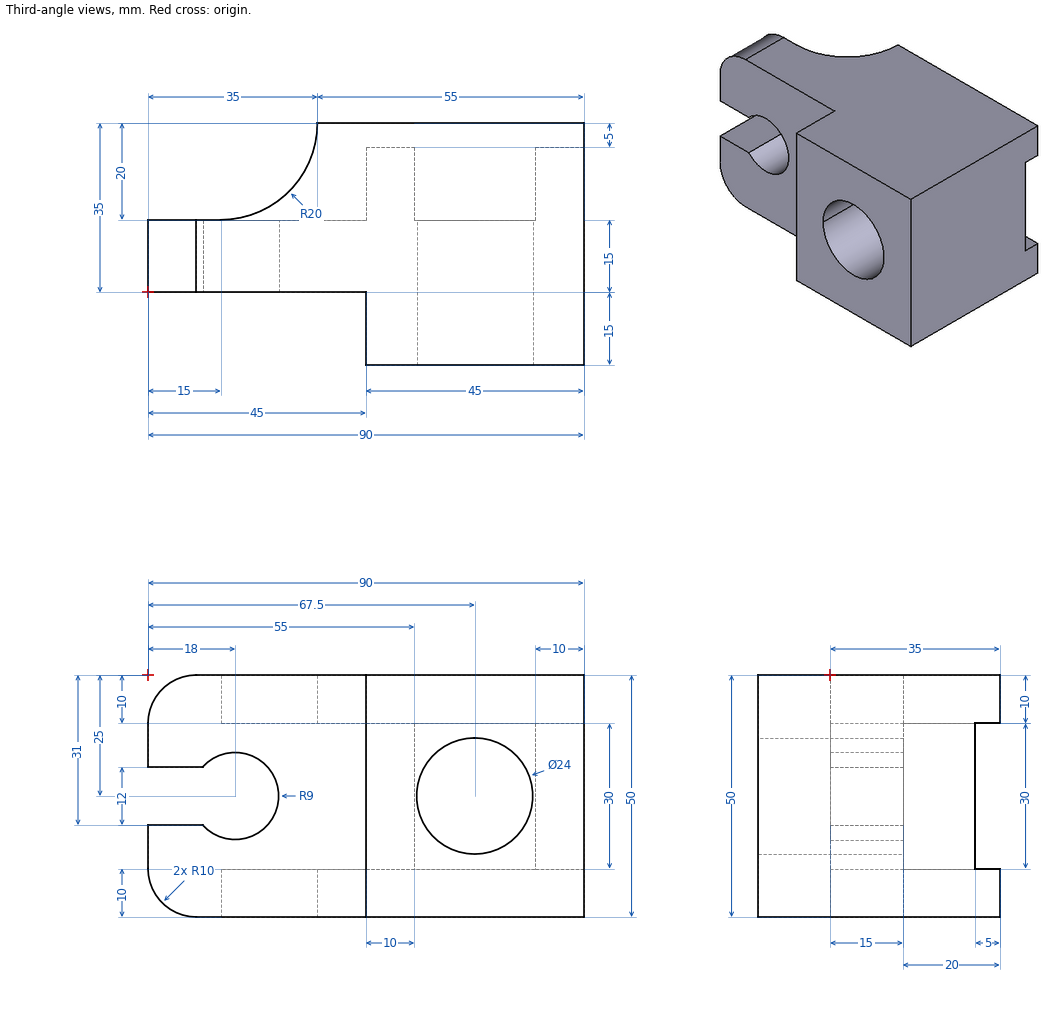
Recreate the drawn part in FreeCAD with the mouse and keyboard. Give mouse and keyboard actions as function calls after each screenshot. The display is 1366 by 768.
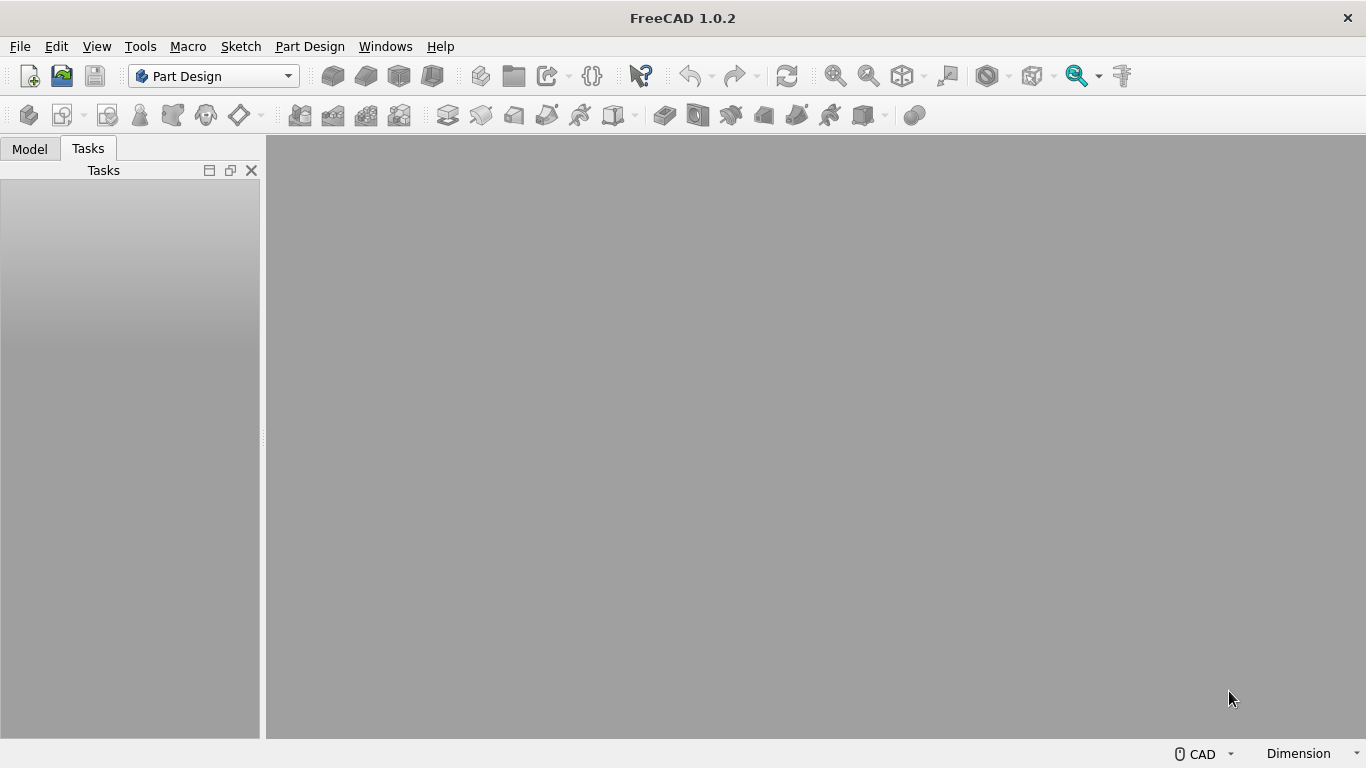
click(29, 76)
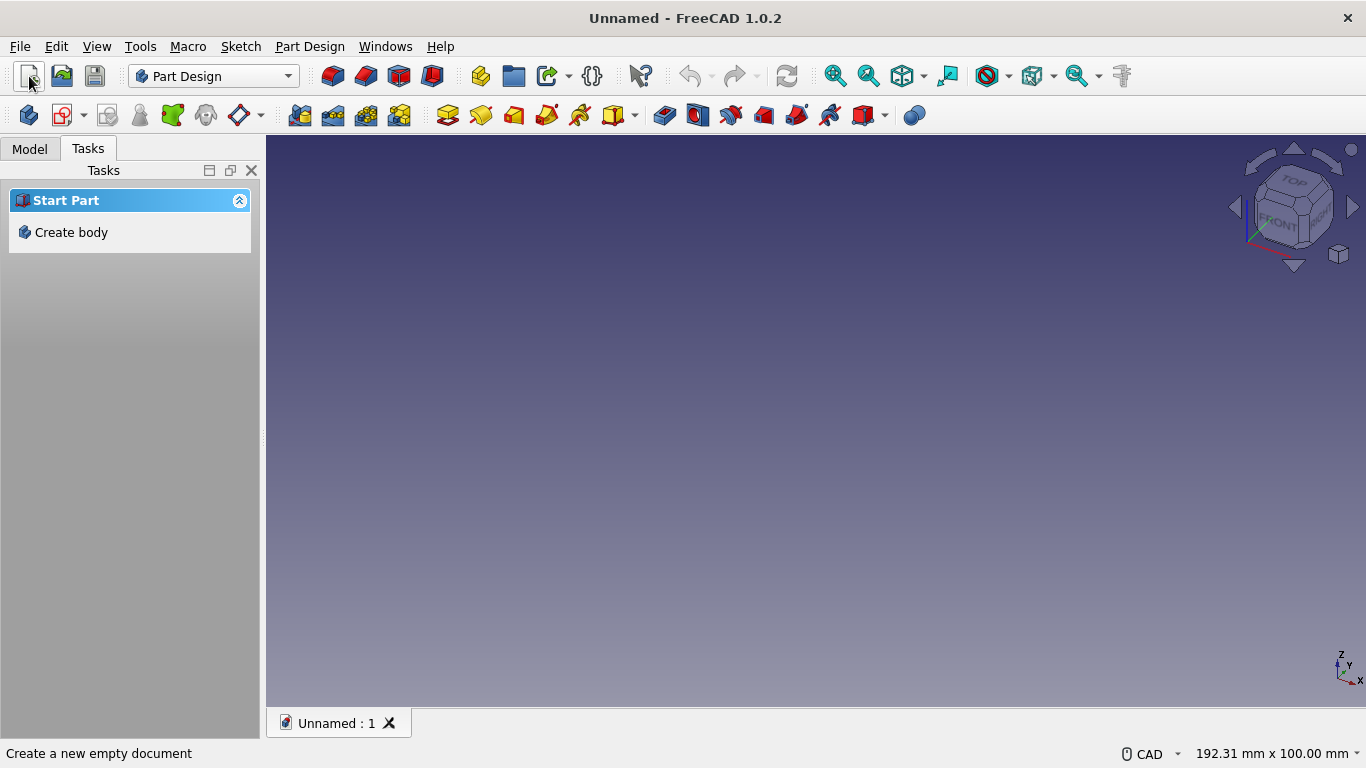
click(62, 116)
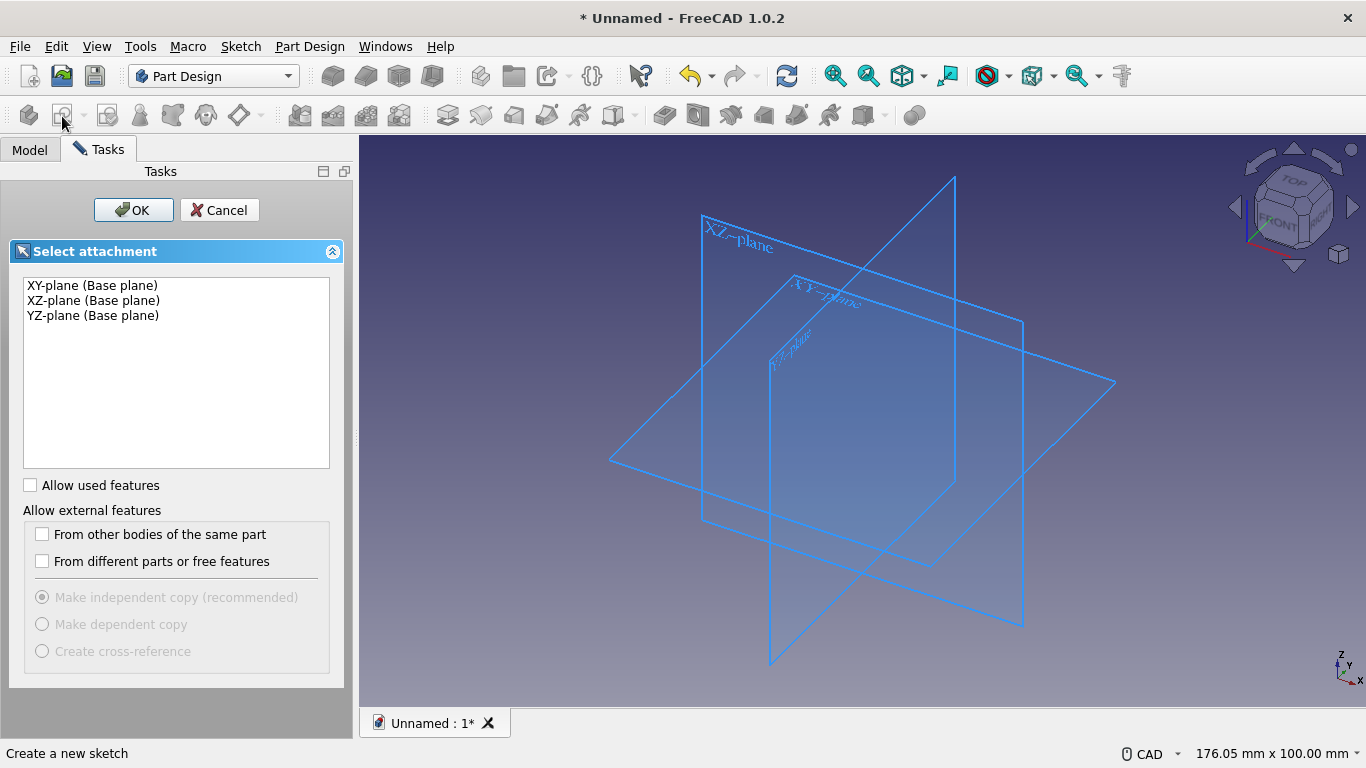
click(84, 286)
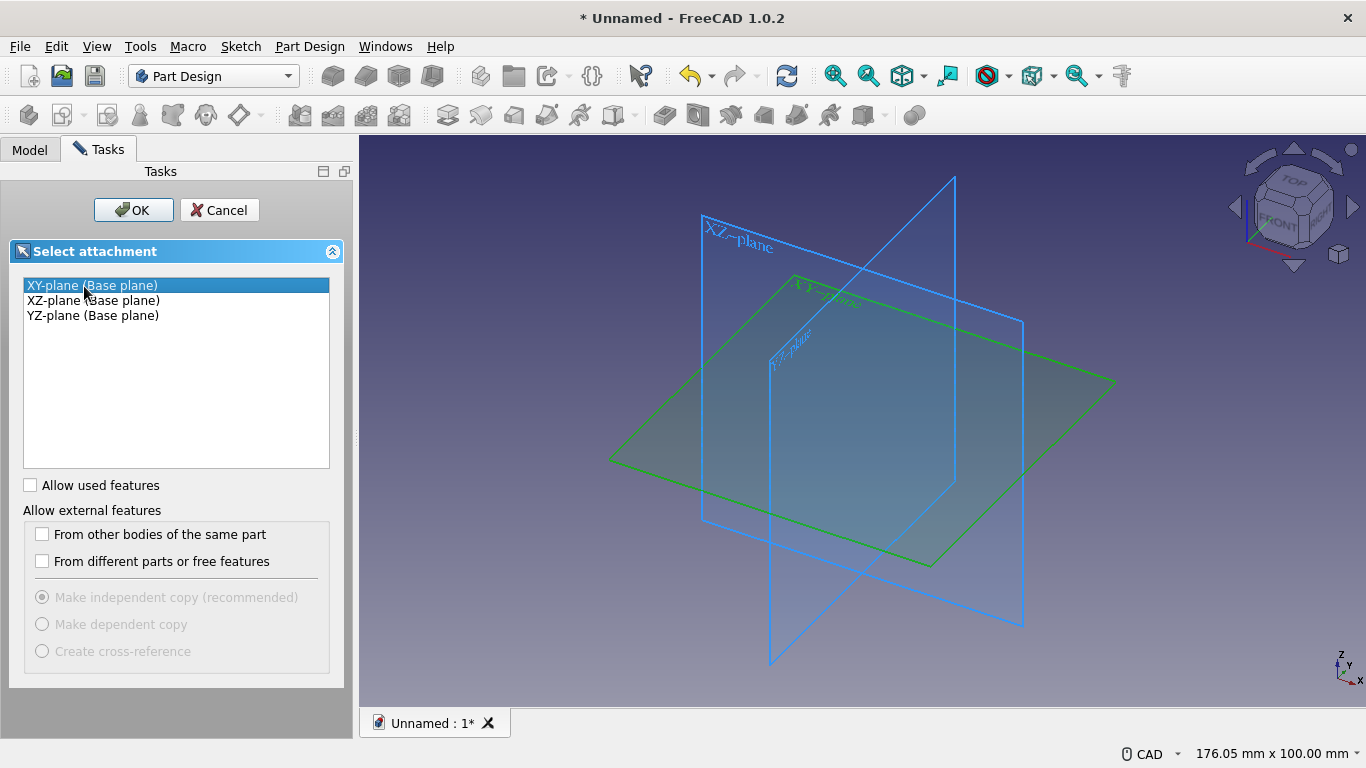
click(134, 210)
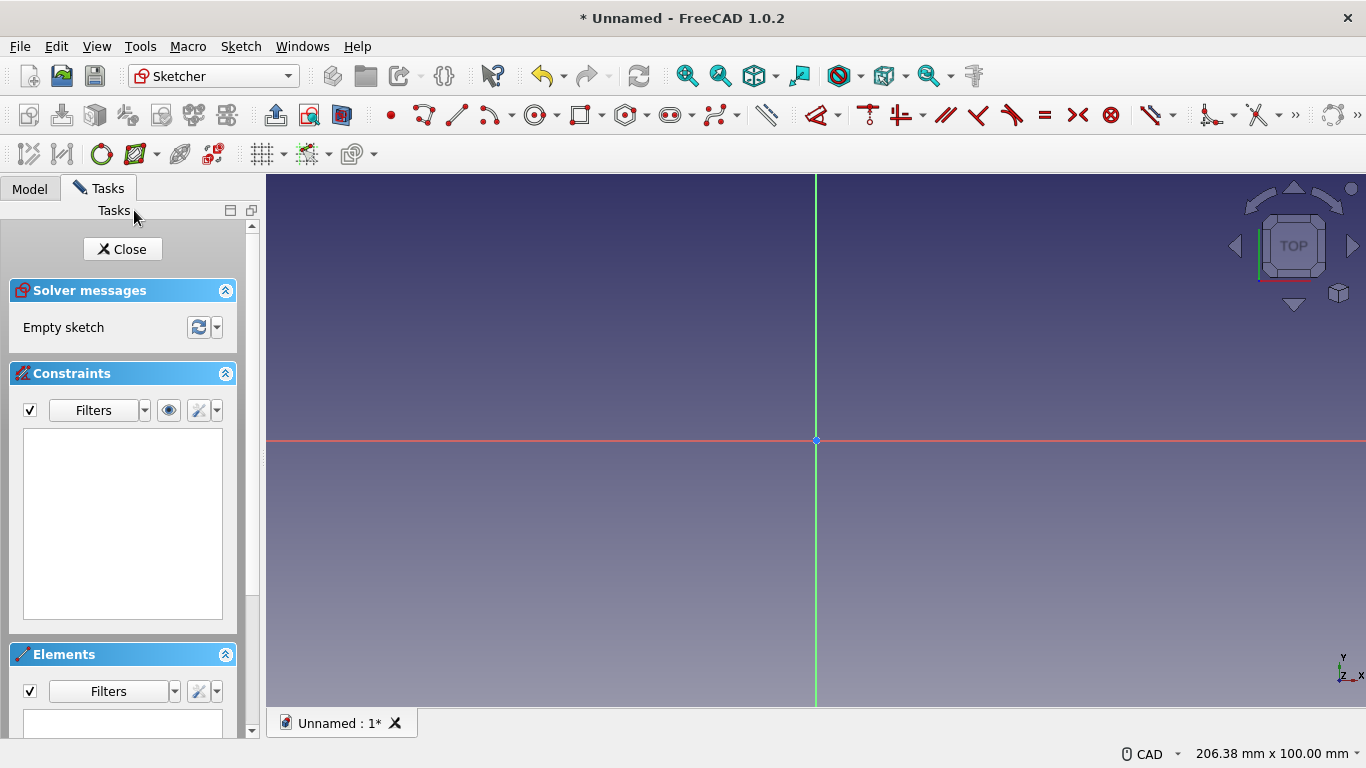
scroll(294, 621, down, 1)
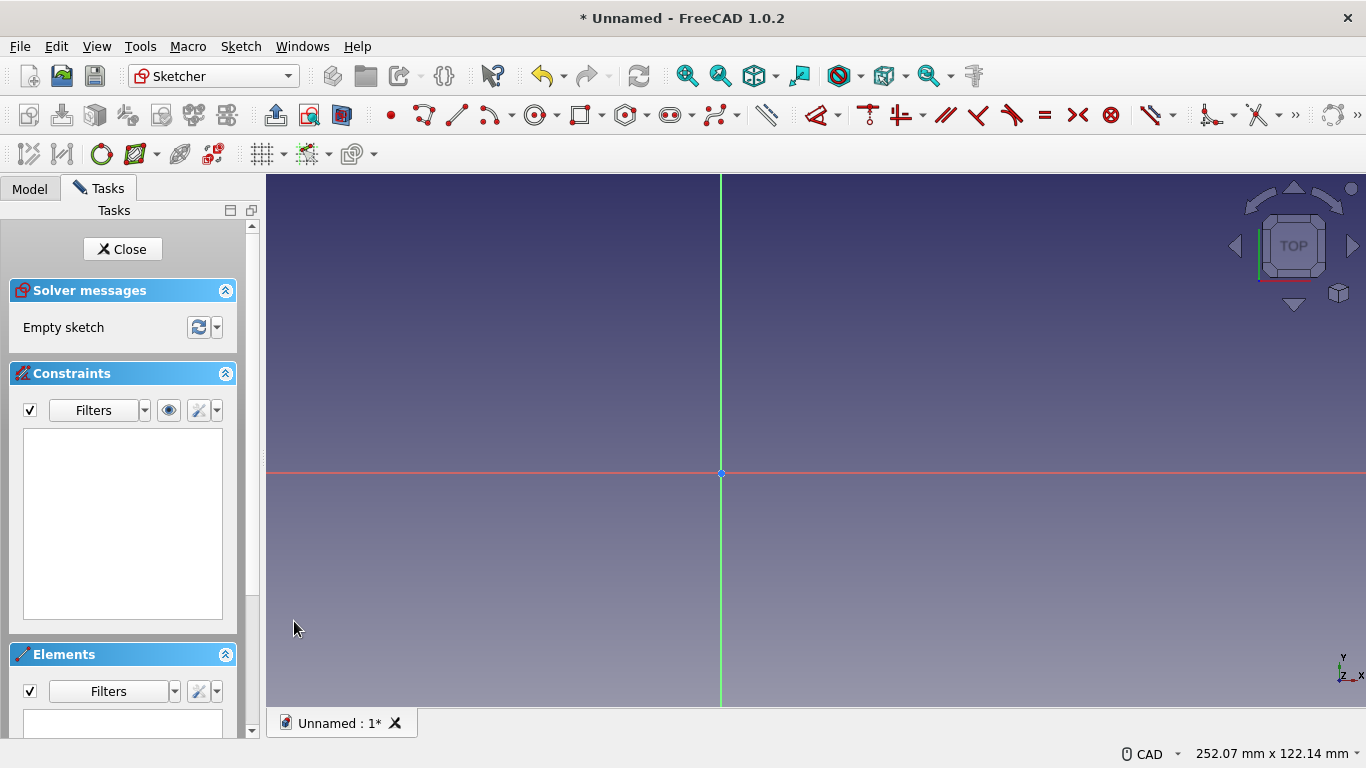
scroll(1201, 441, up, 2)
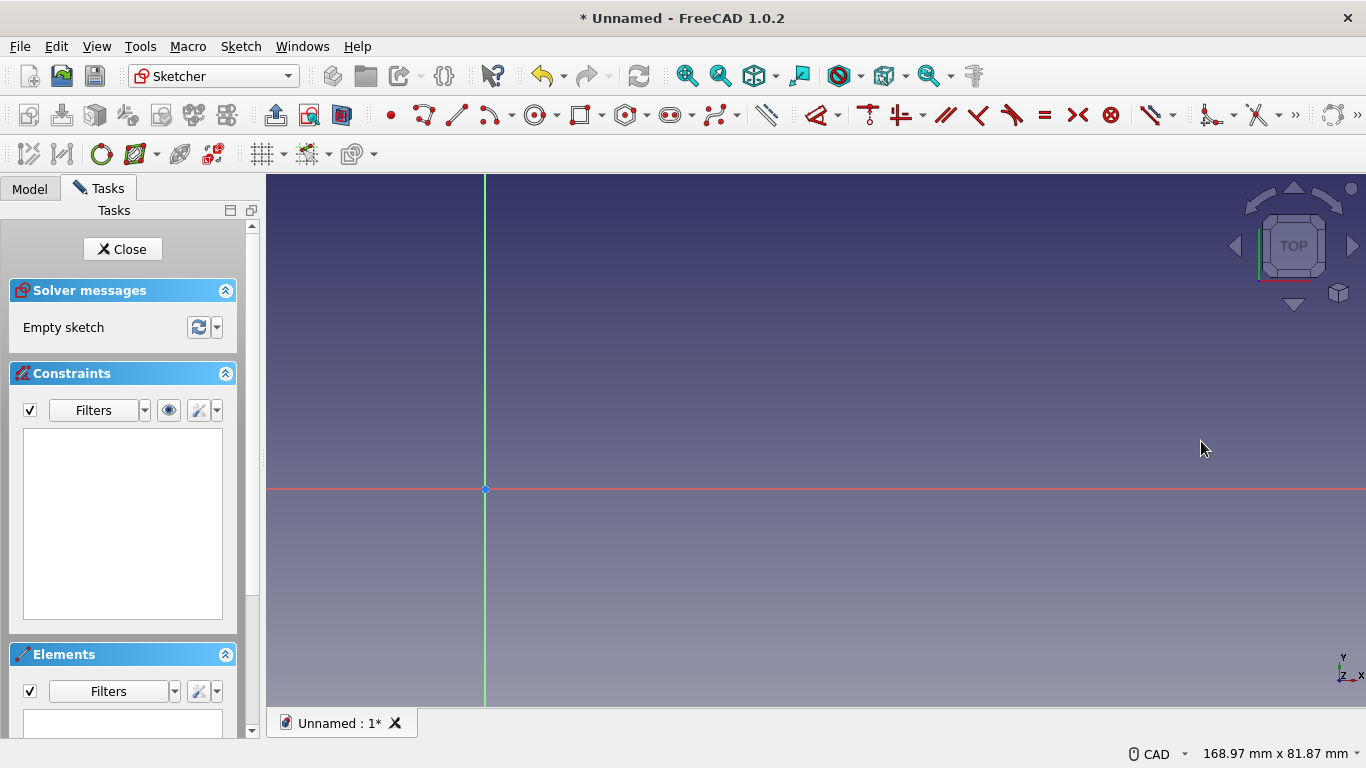
click(580, 116)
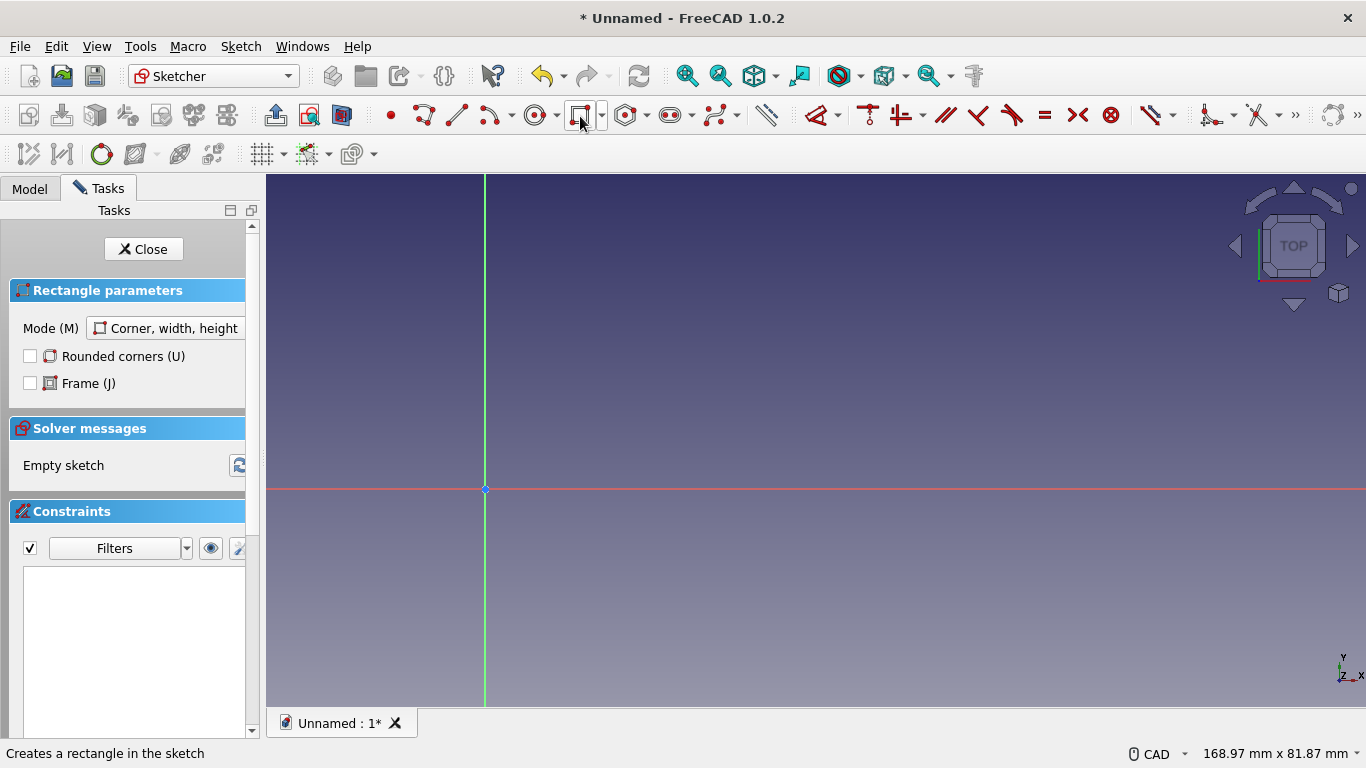
click(485, 489)
click(1071, 391)
key(Escape)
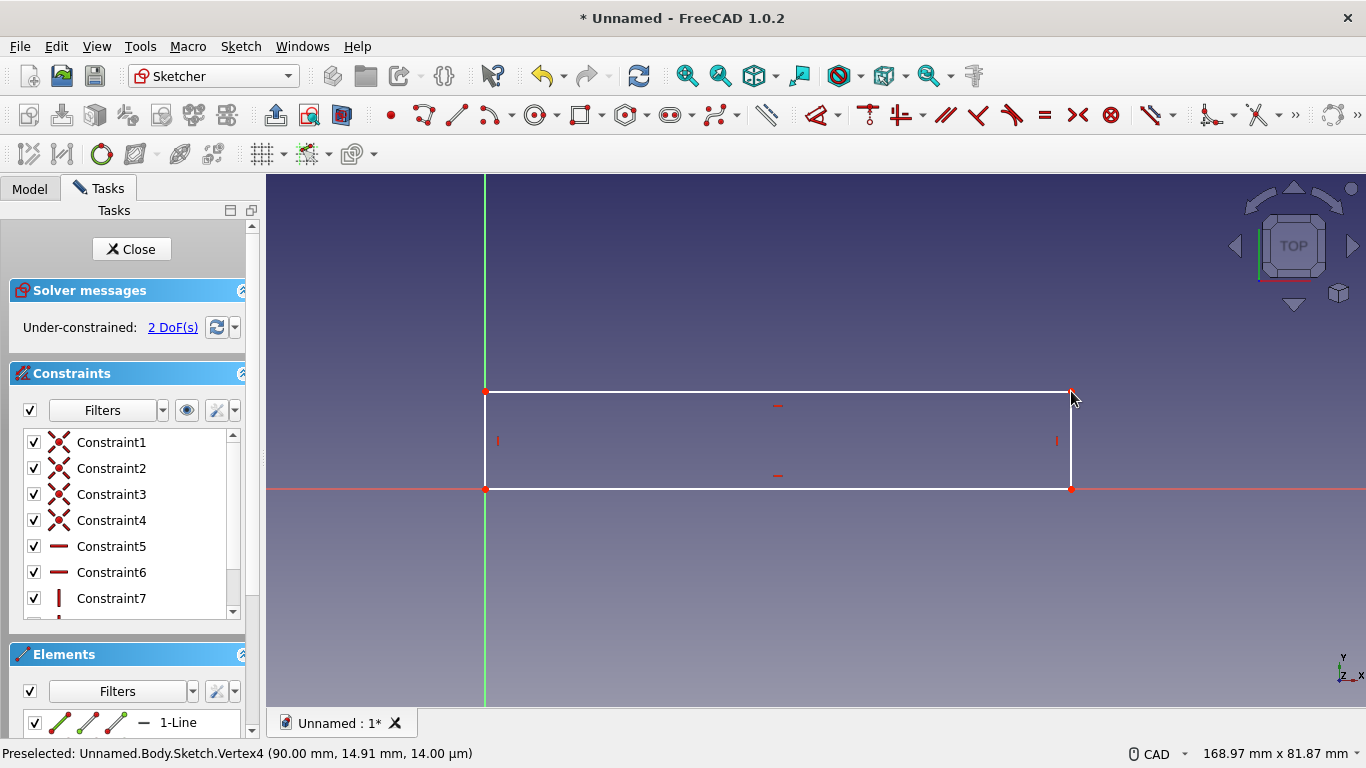
key(d)